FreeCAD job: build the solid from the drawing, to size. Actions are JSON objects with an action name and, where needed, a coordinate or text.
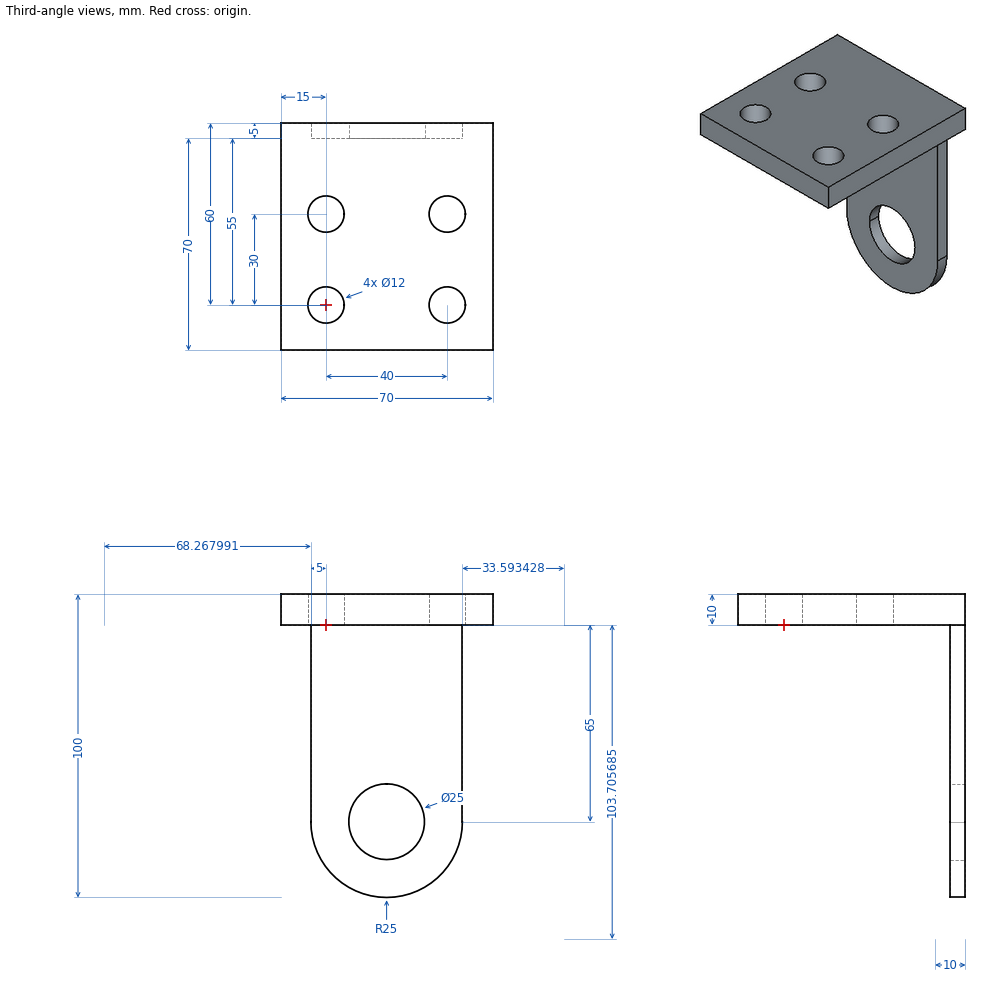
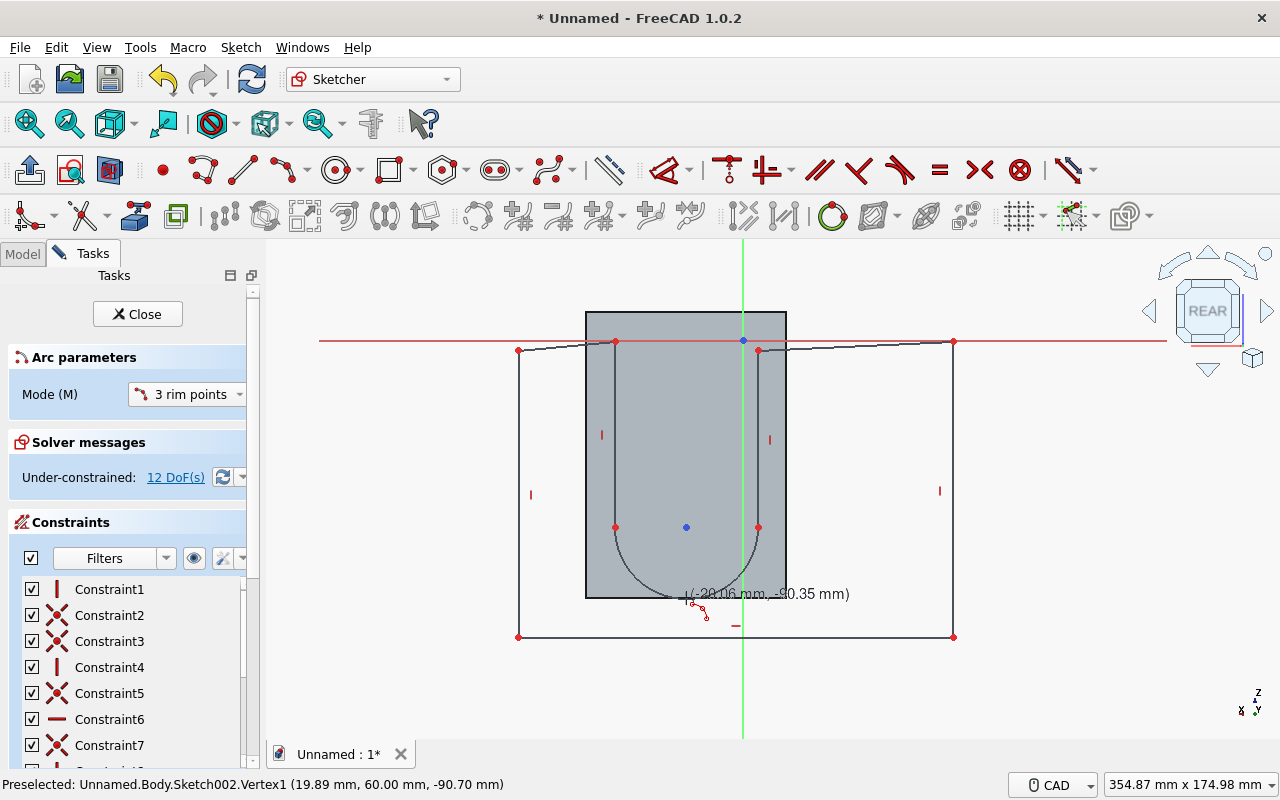
{"action": "left_click", "coordinate": [336, 170]}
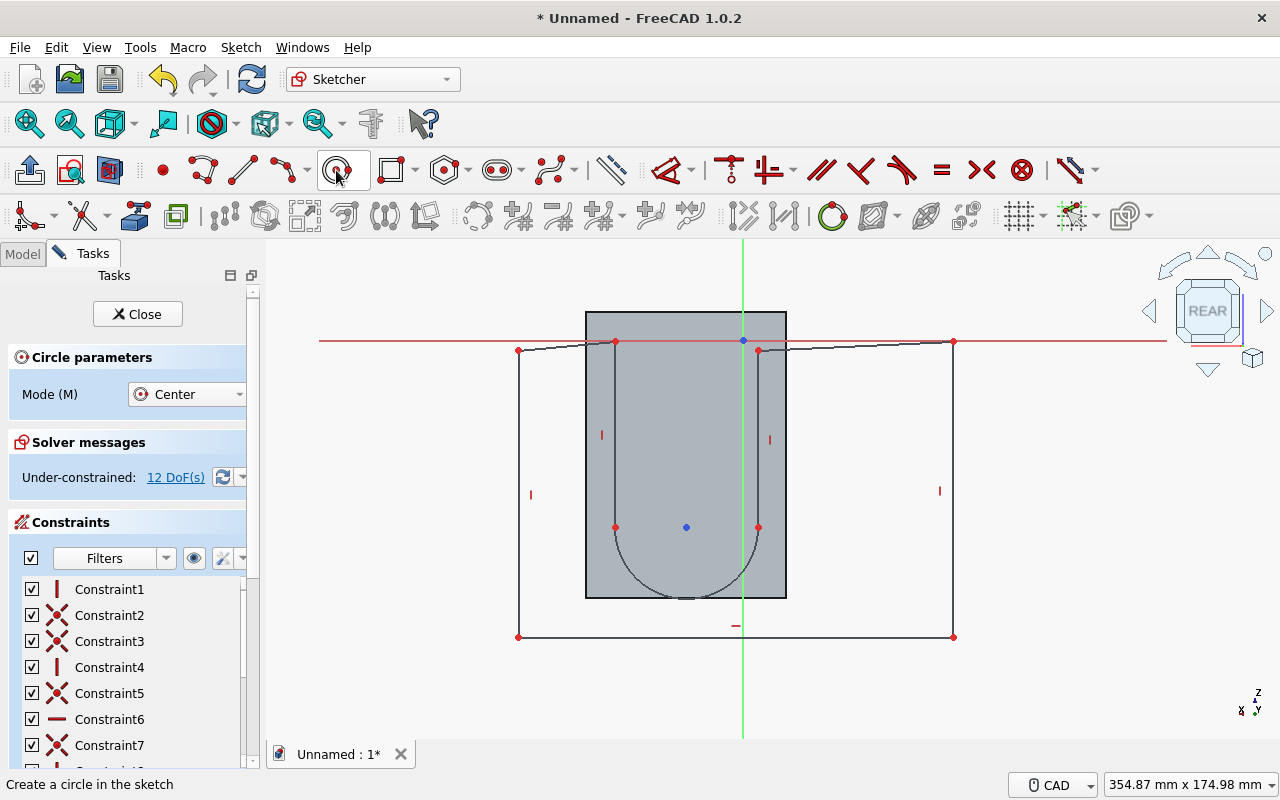
{"action": "left_click", "coordinate": [686, 527]}
{"action": "left_click", "coordinate": [711, 501]}
{"action": "key", "text": "Escape"}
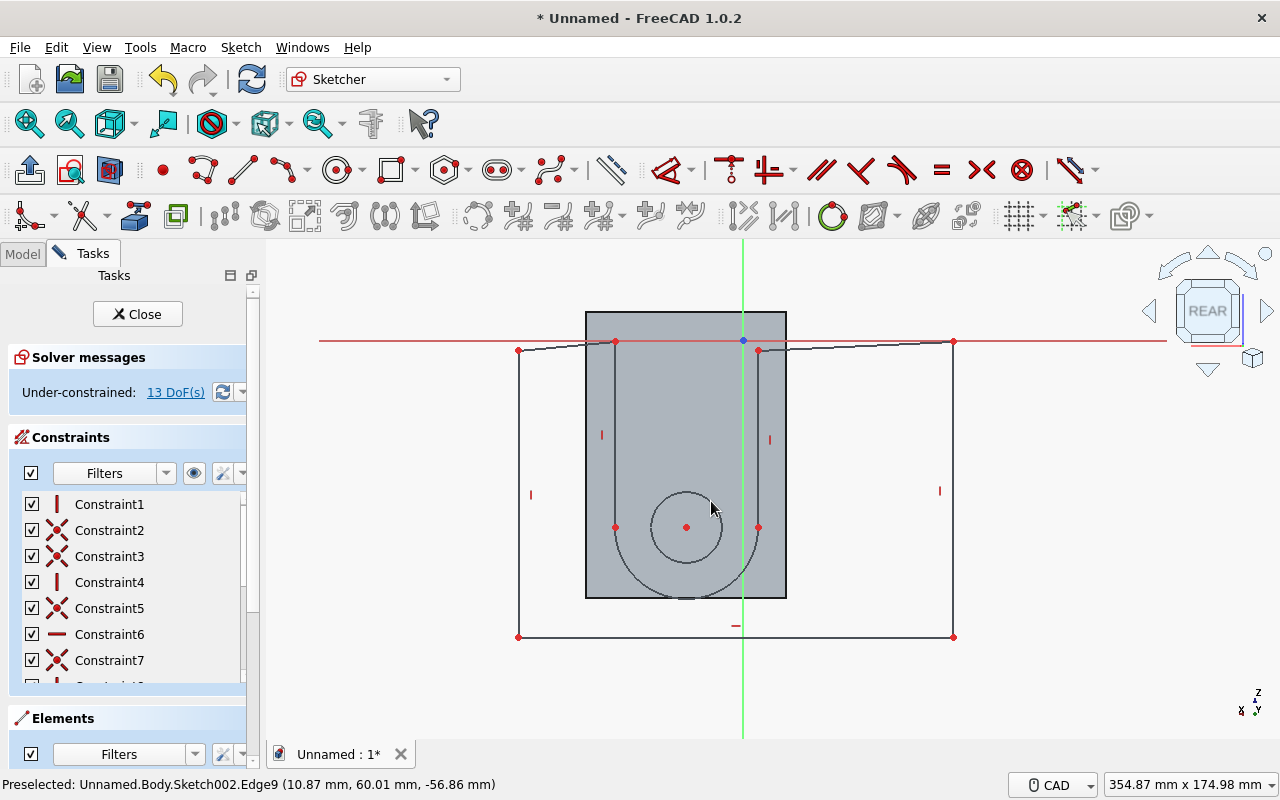
{"action": "left_click", "coordinate": [615, 472]}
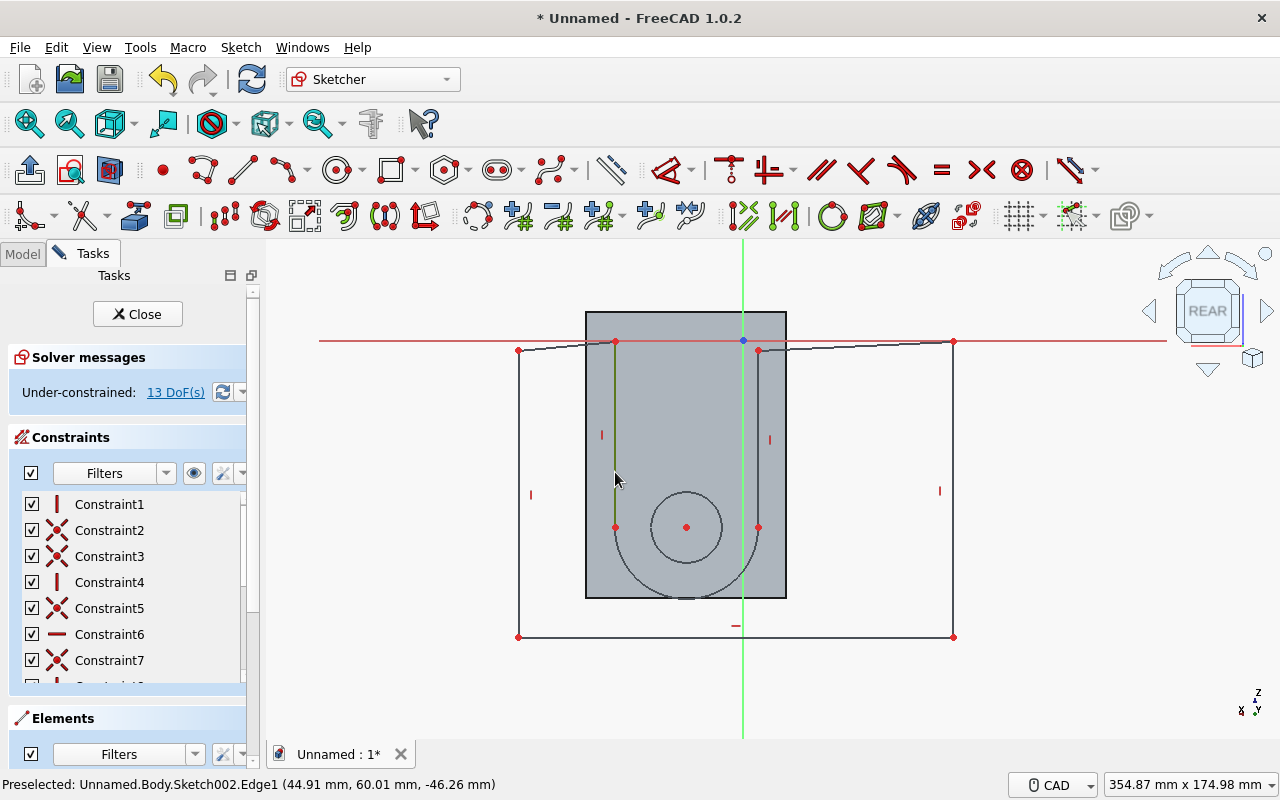
{"action": "left_click", "coordinate": [645, 585]}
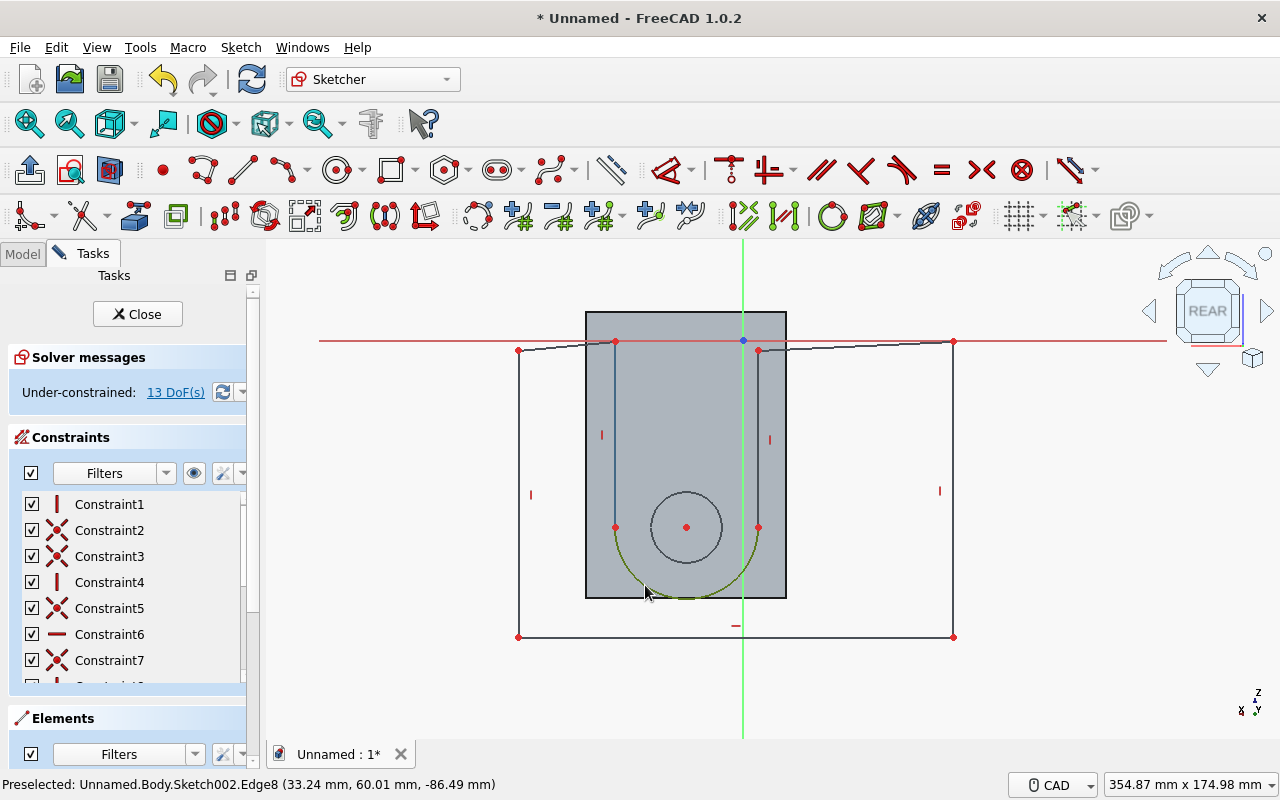
{"action": "left_click", "coordinate": [902, 170]}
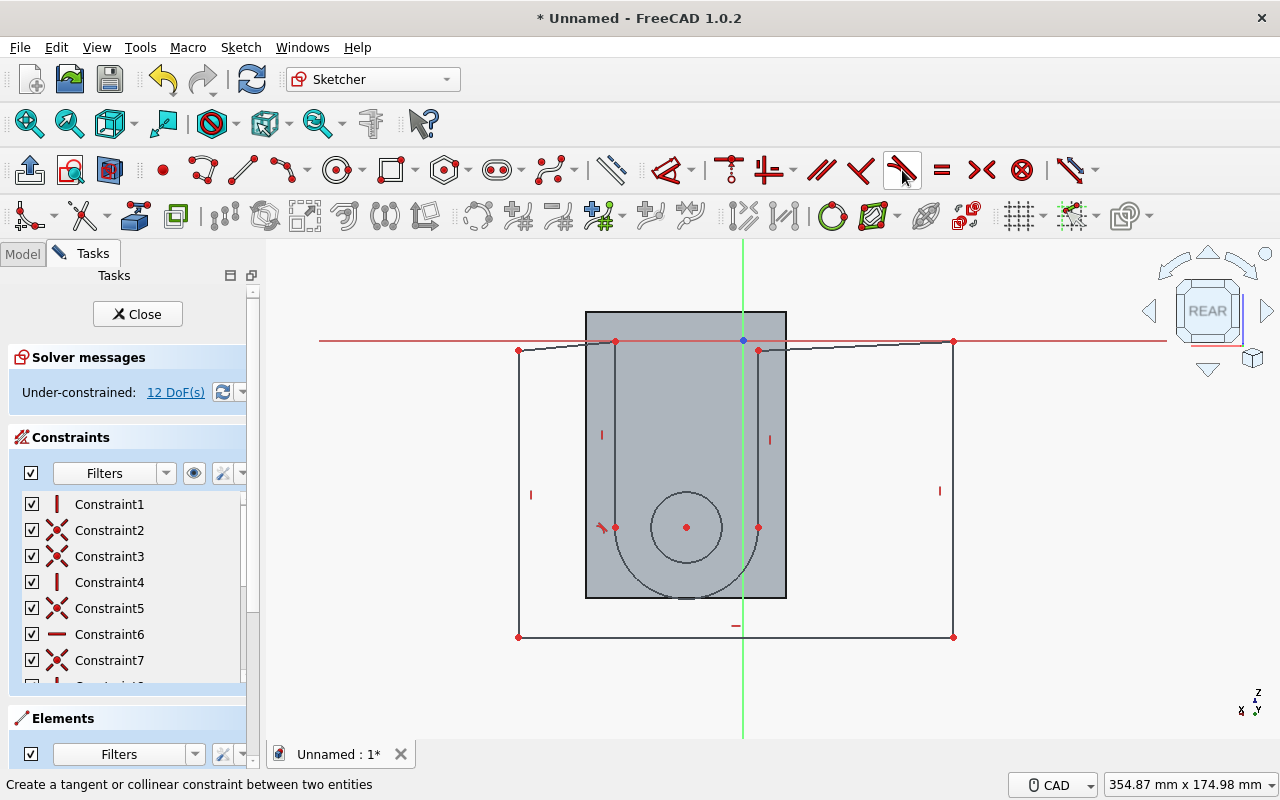
{"action": "left_click", "coordinate": [758, 404]}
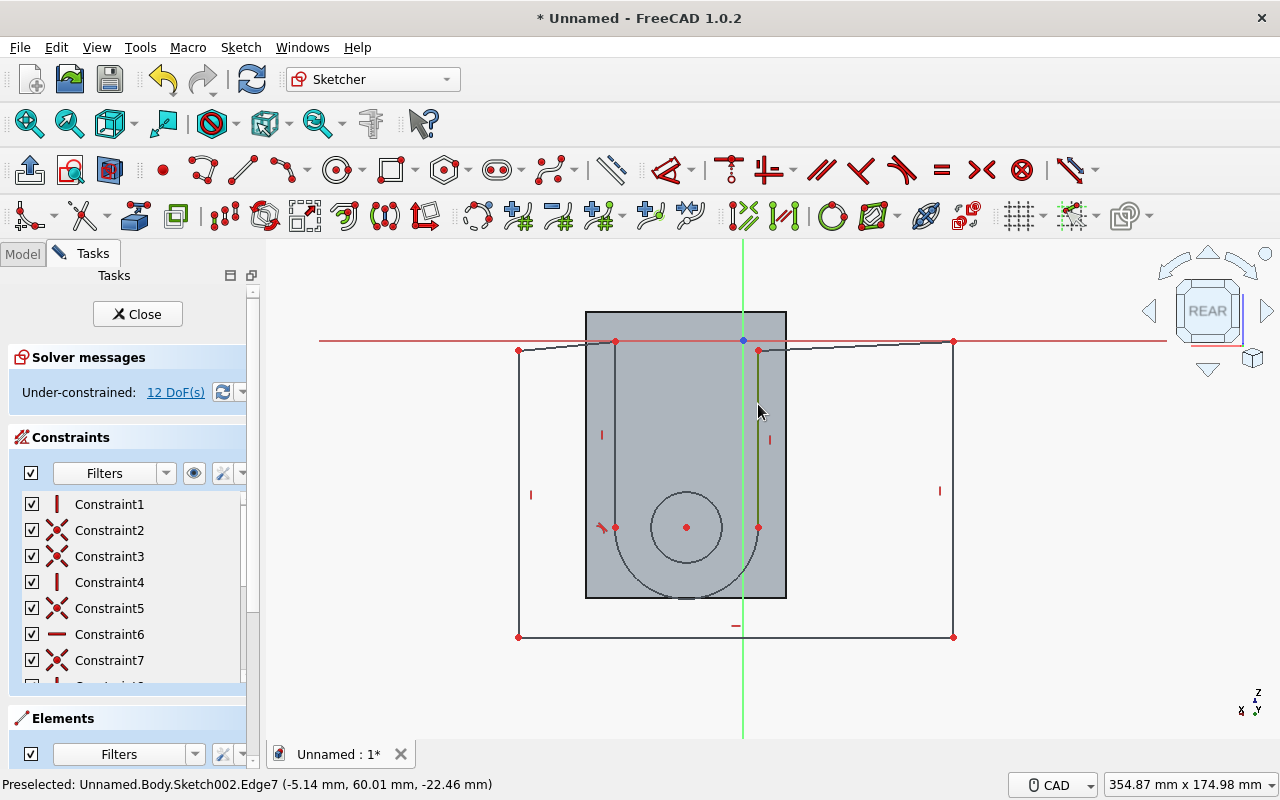
{"action": "left_click", "coordinate": [644, 585]}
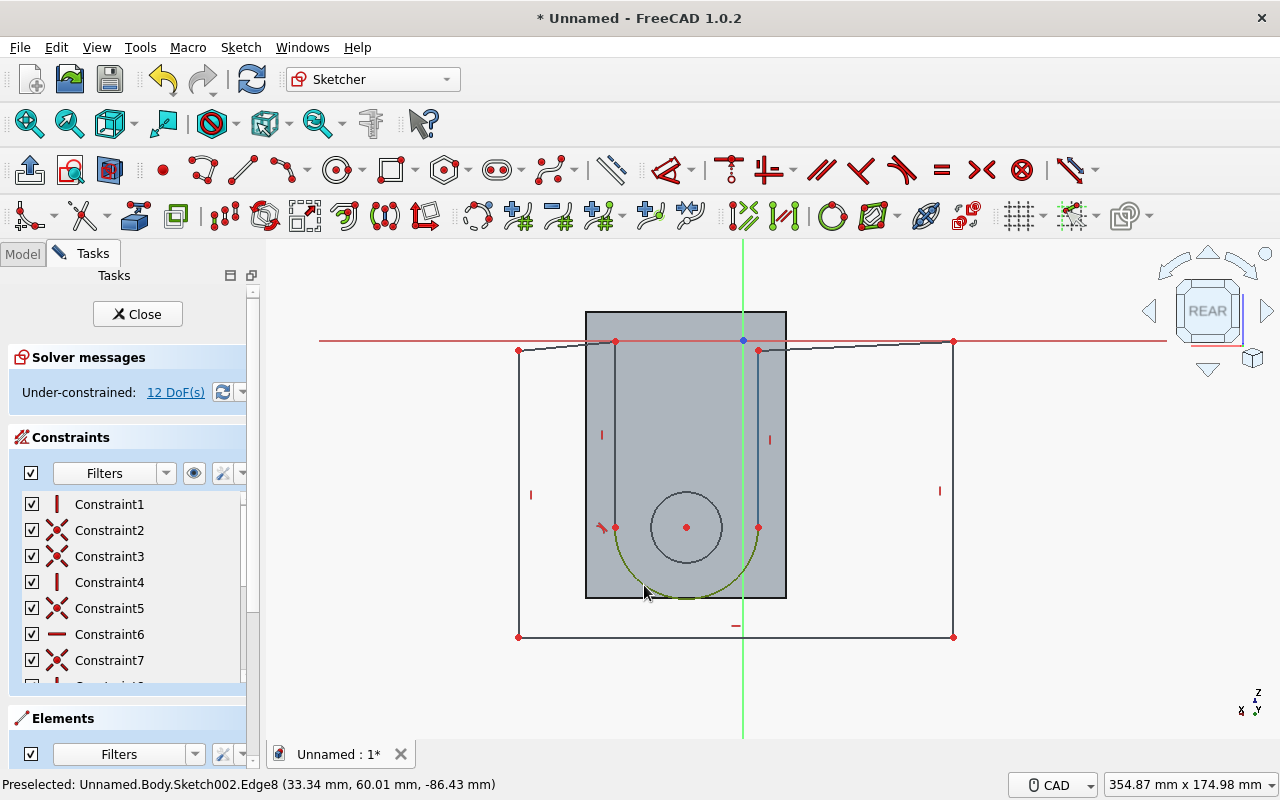
{"action": "left_click", "coordinate": [902, 170]}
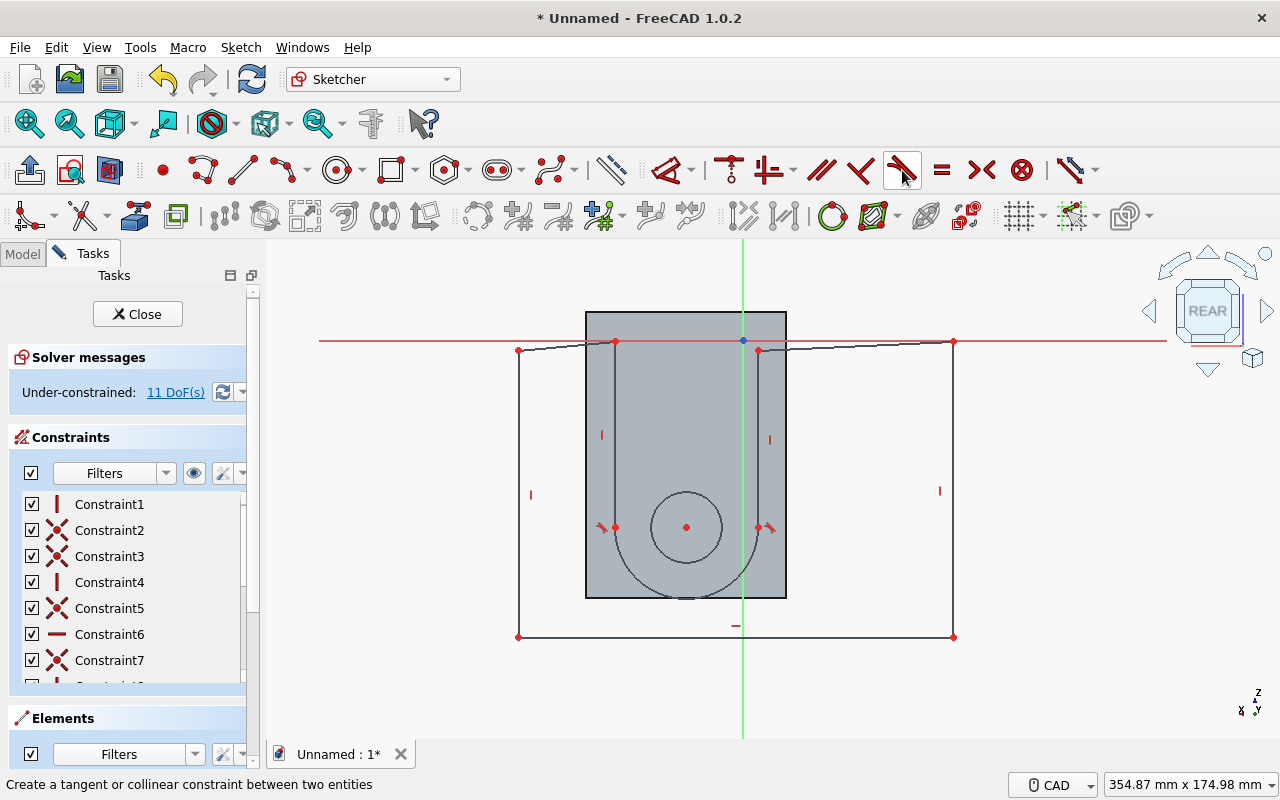
{"action": "left_click", "coordinate": [586, 345]}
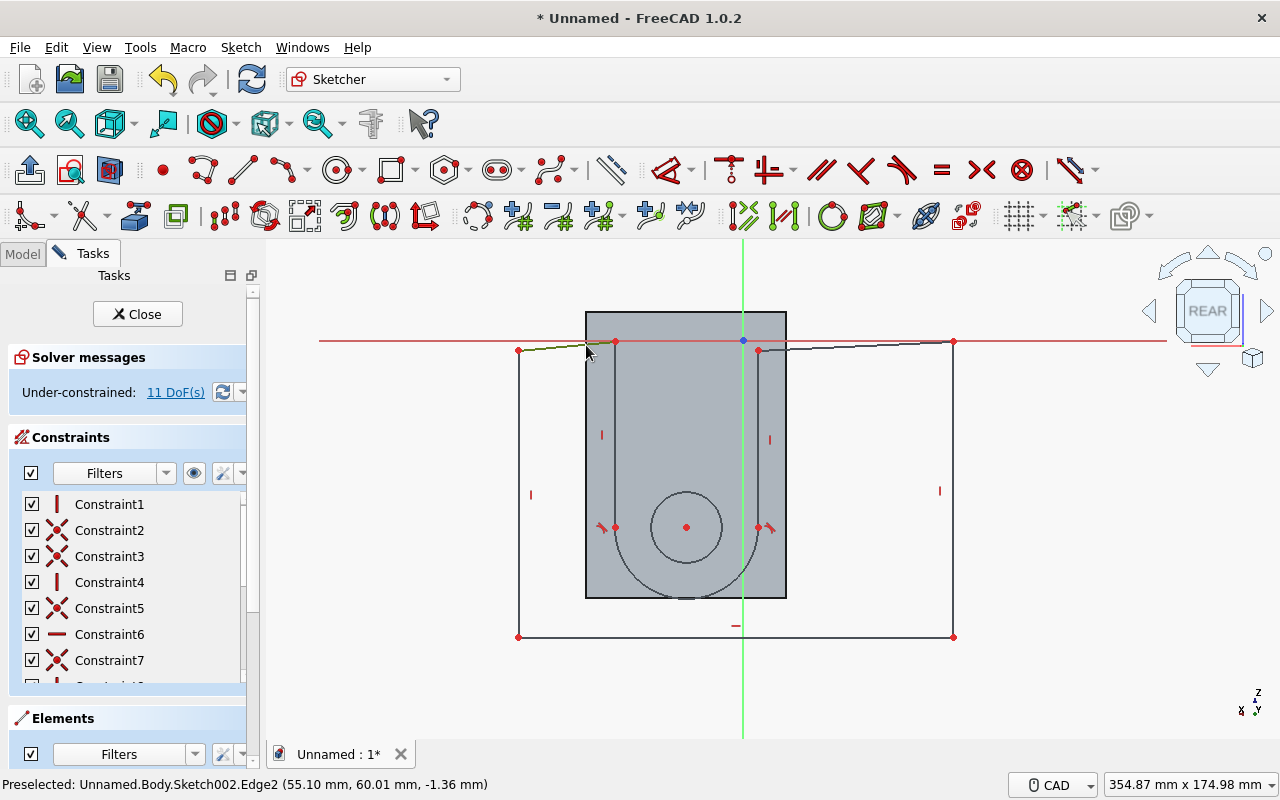
{"action": "left_click", "coordinate": [796, 170]}